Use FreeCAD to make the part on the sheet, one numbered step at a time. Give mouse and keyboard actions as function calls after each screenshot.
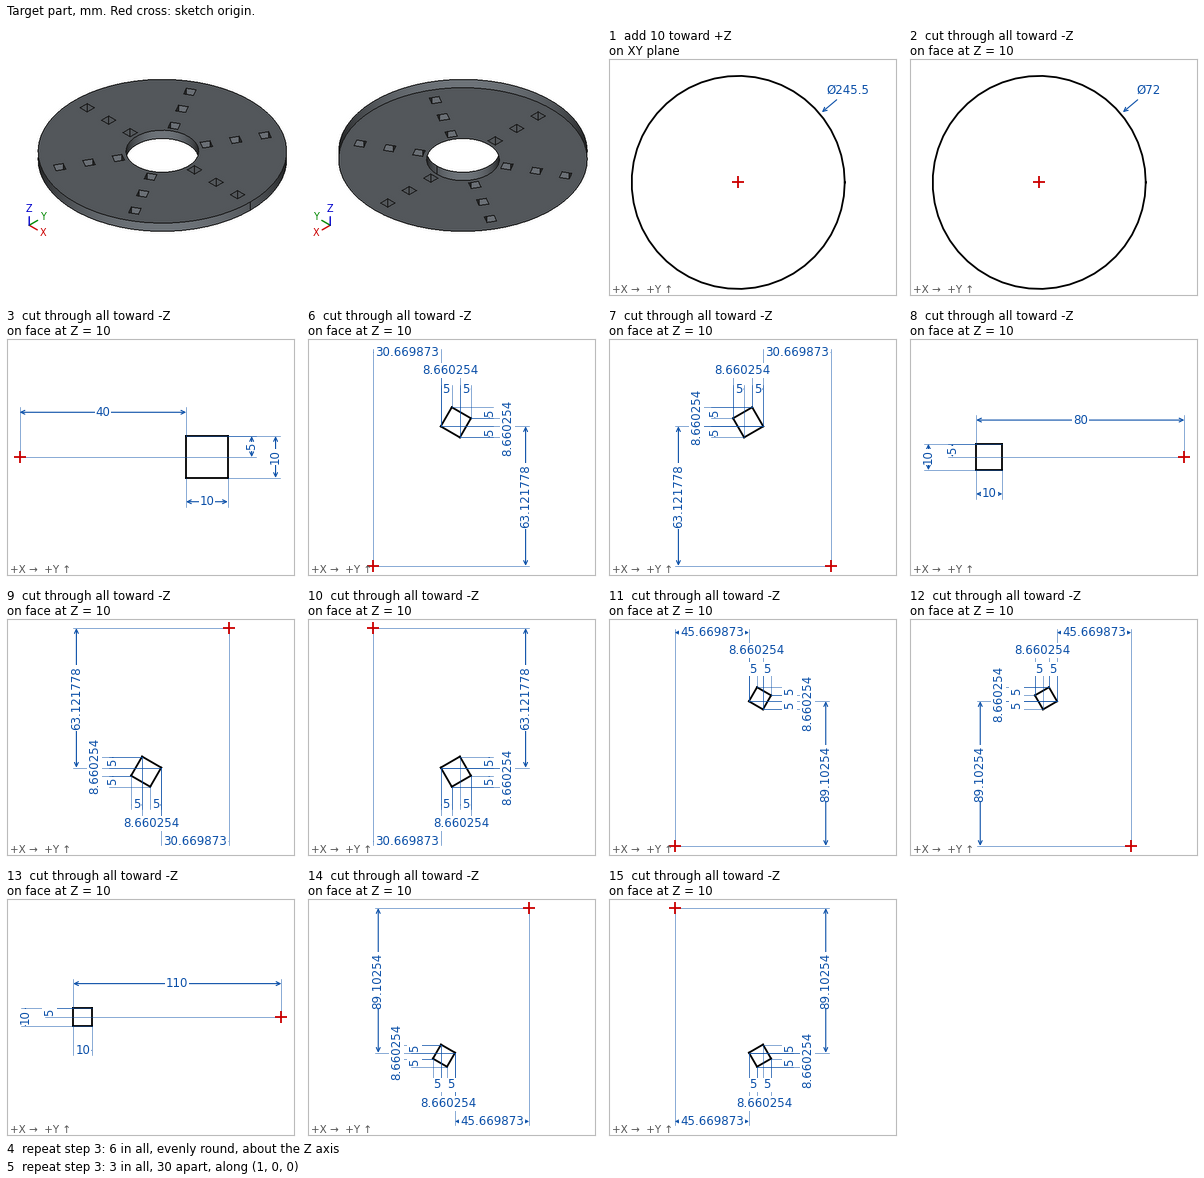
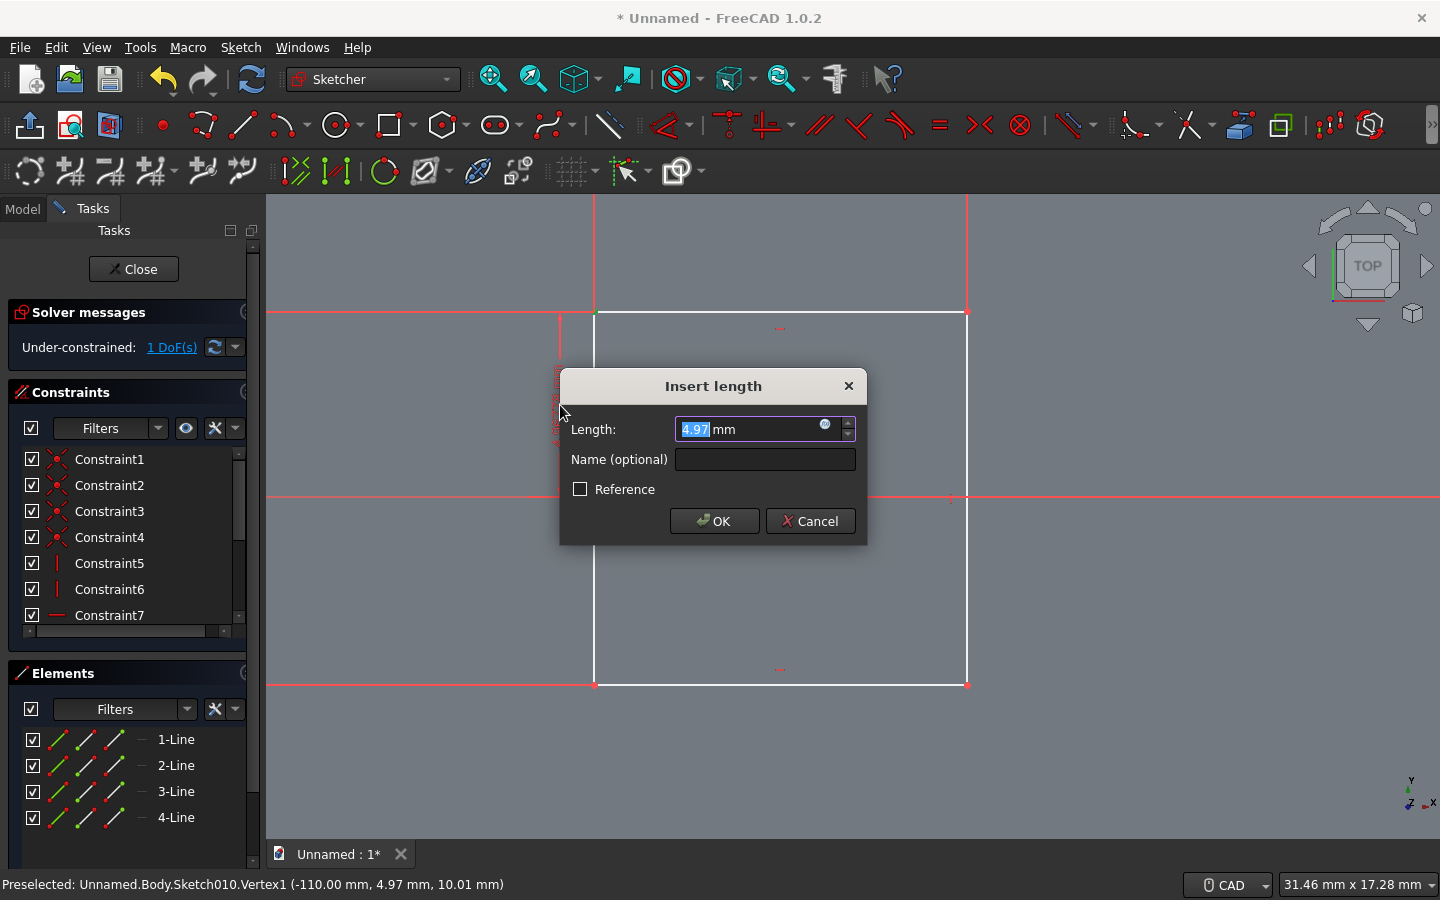
text(5)
key(Return)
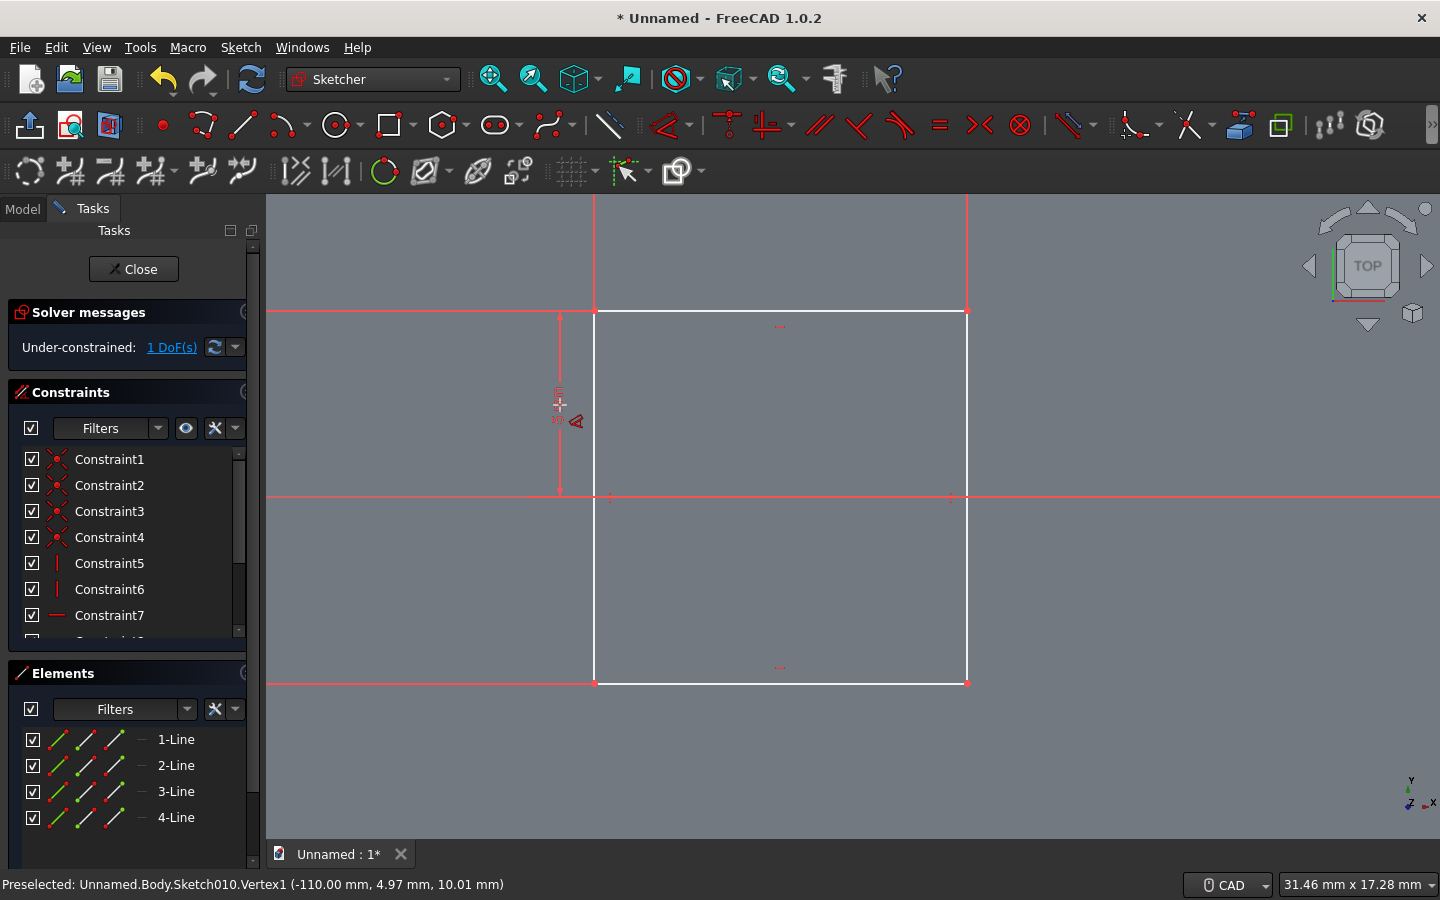
click(594, 311)
click(935, 277)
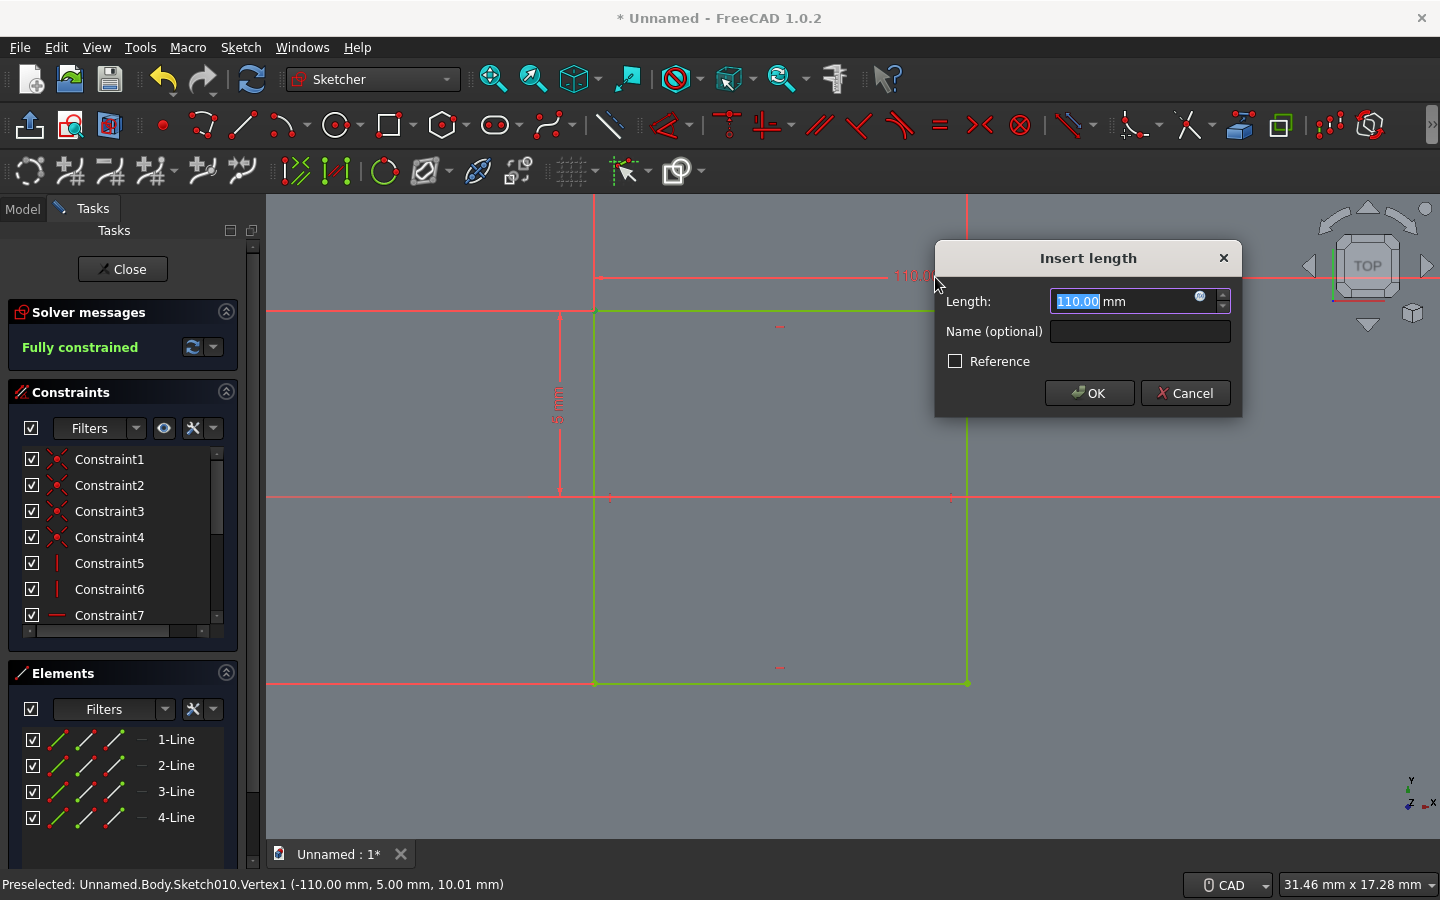
text(110)
key(Return)
key(Escape)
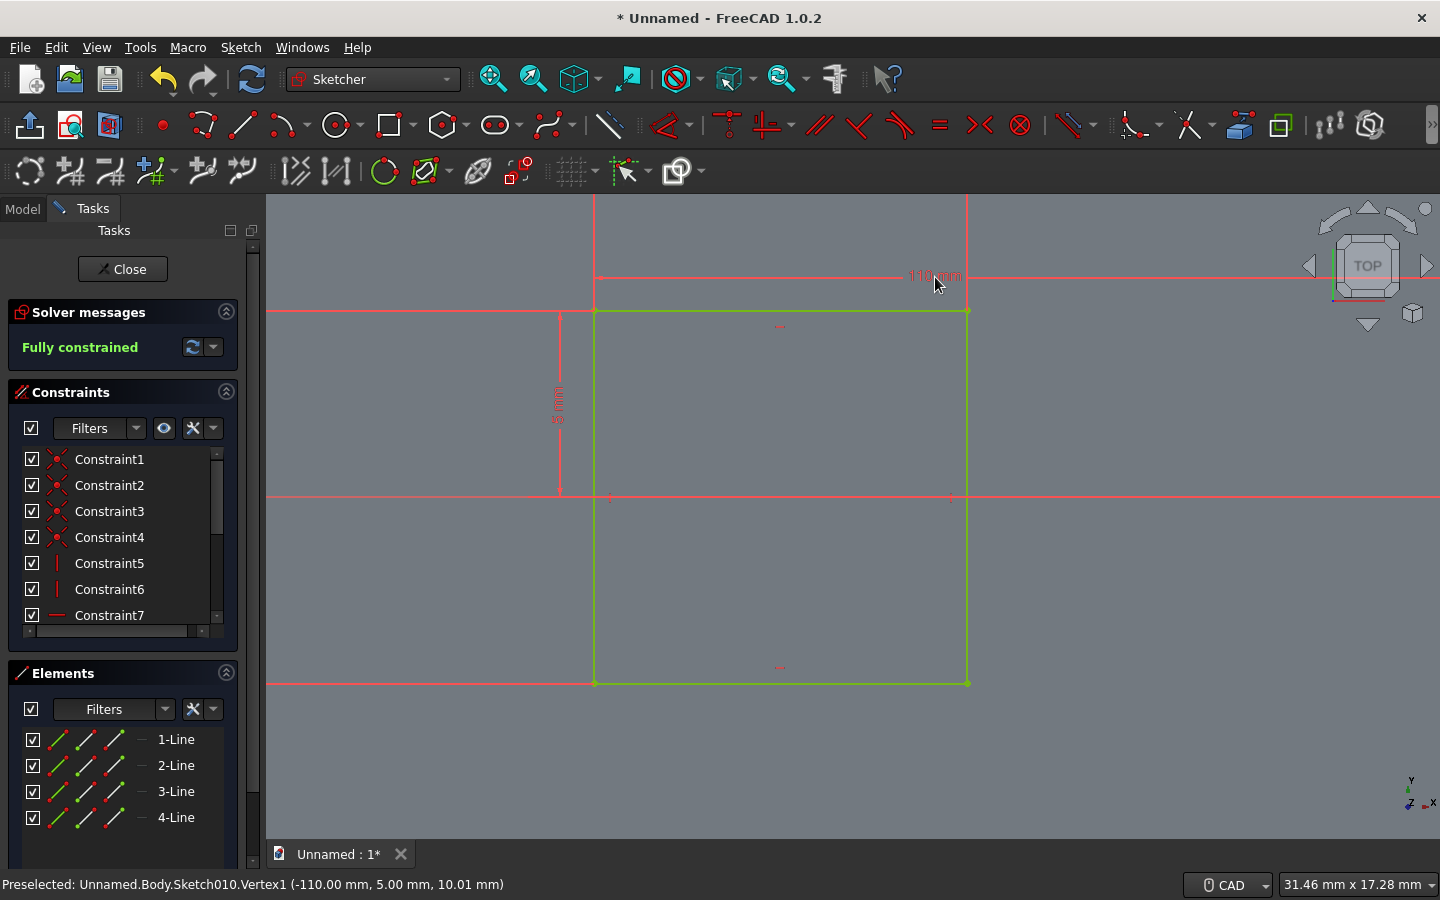
click(123, 269)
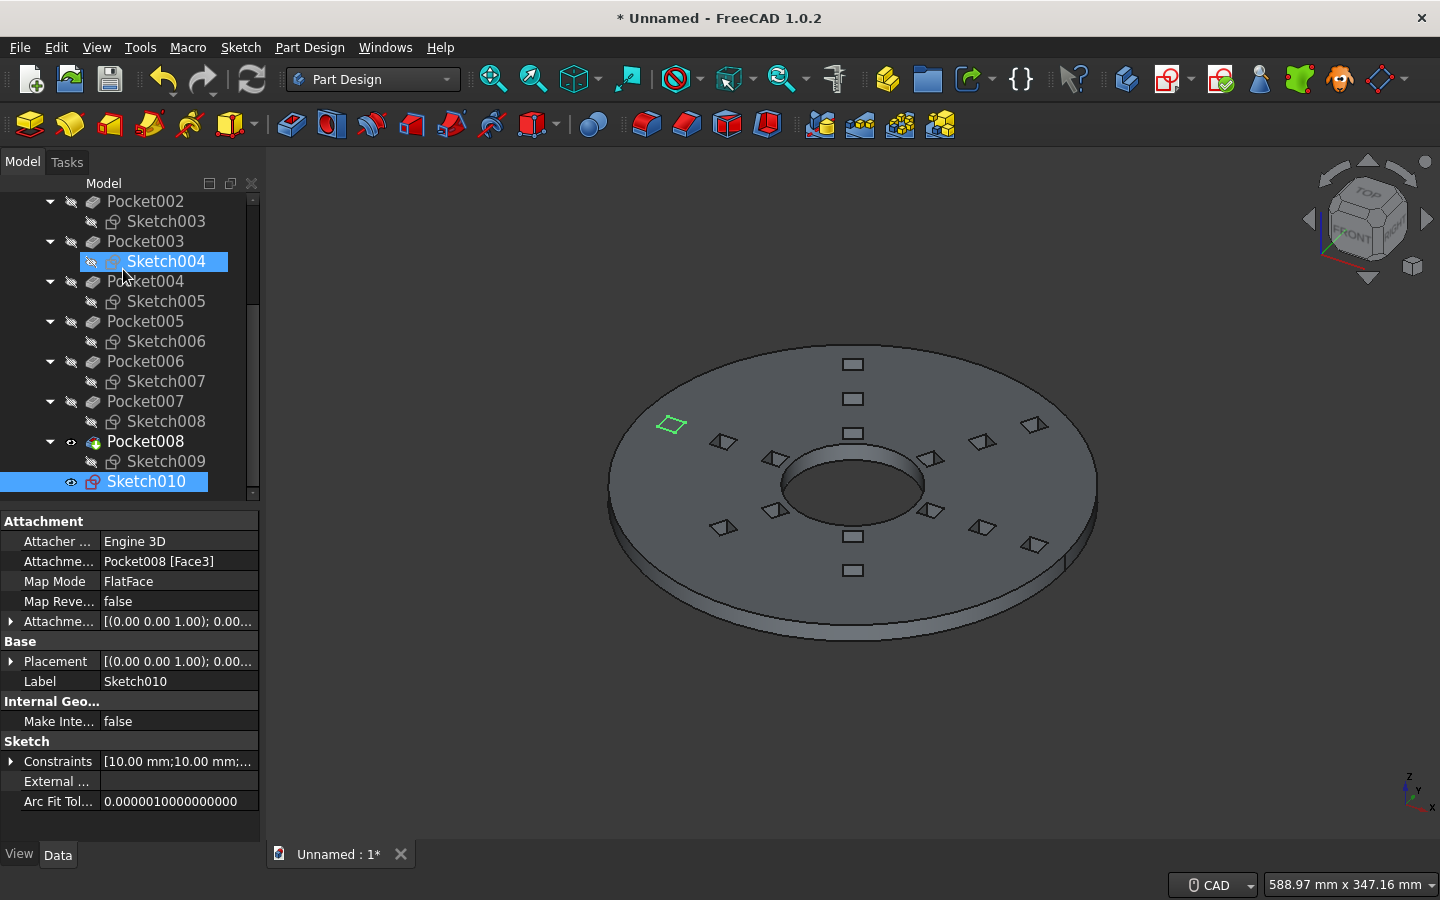
click(292, 124)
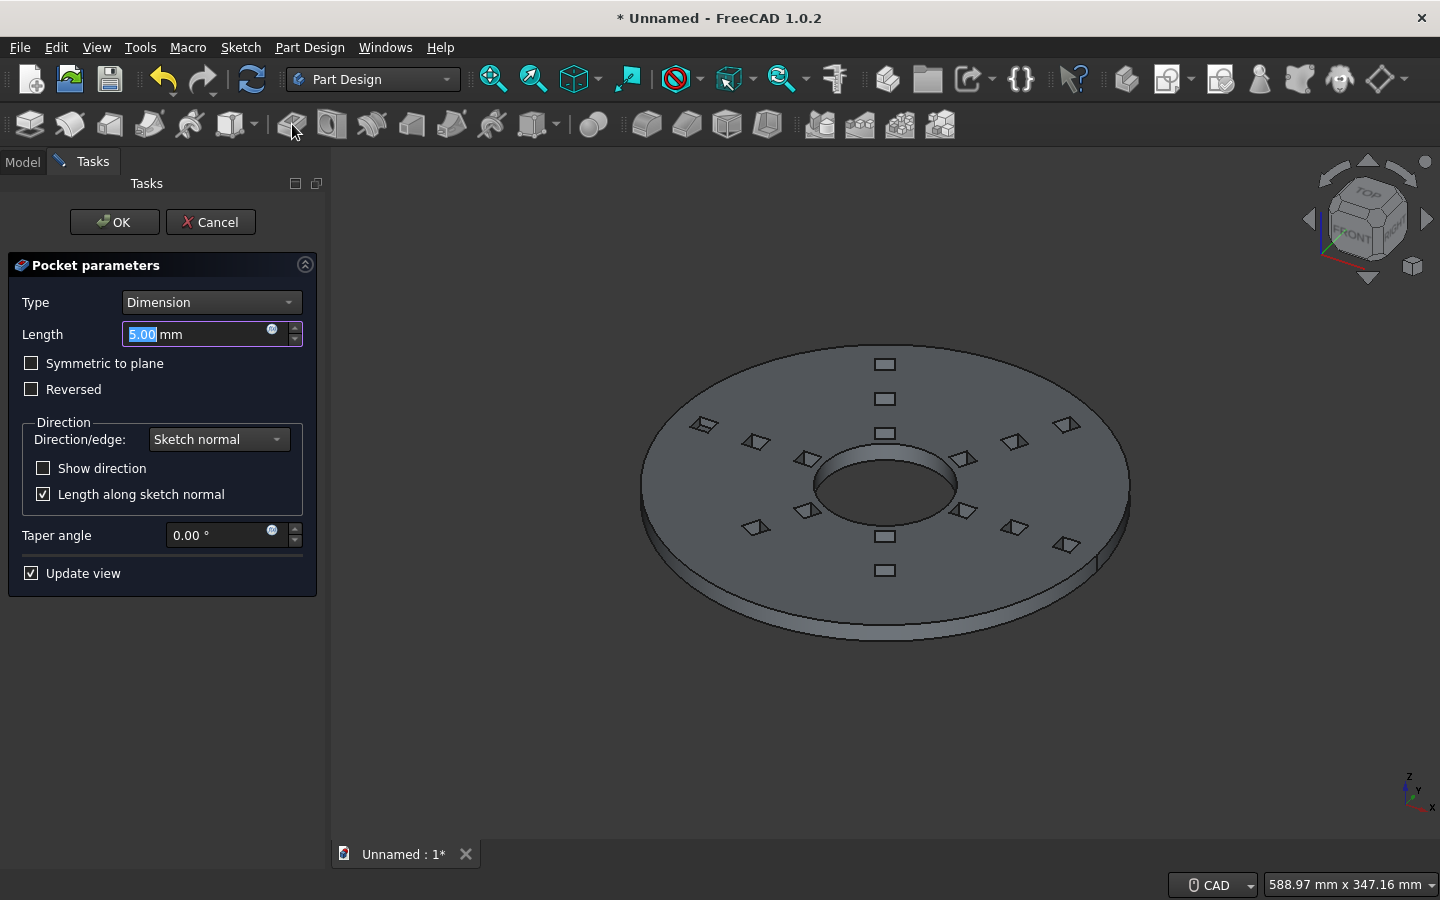
click(212, 302)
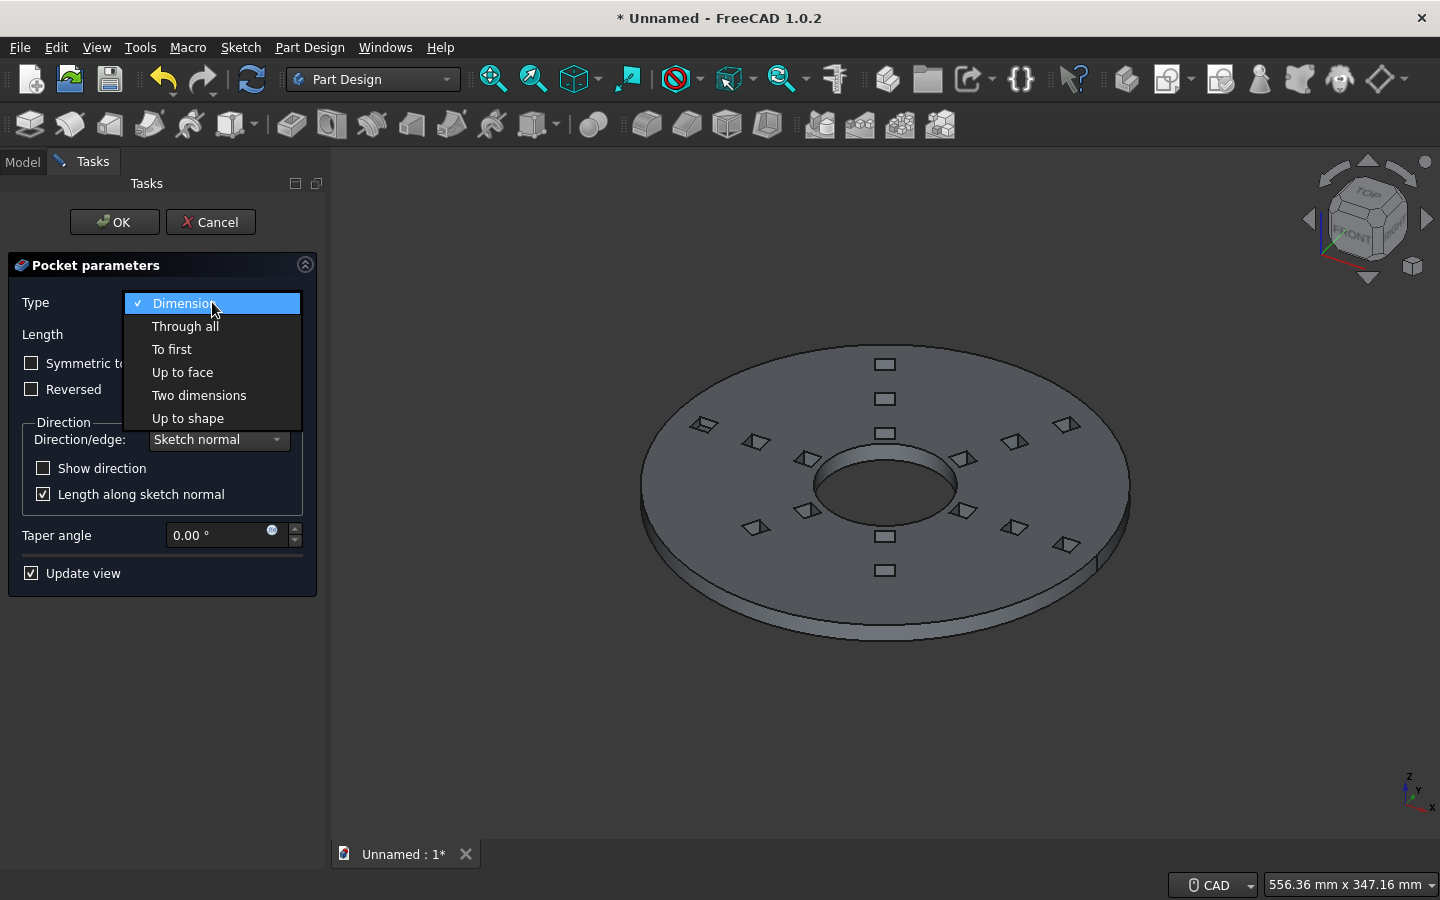
click(212, 326)